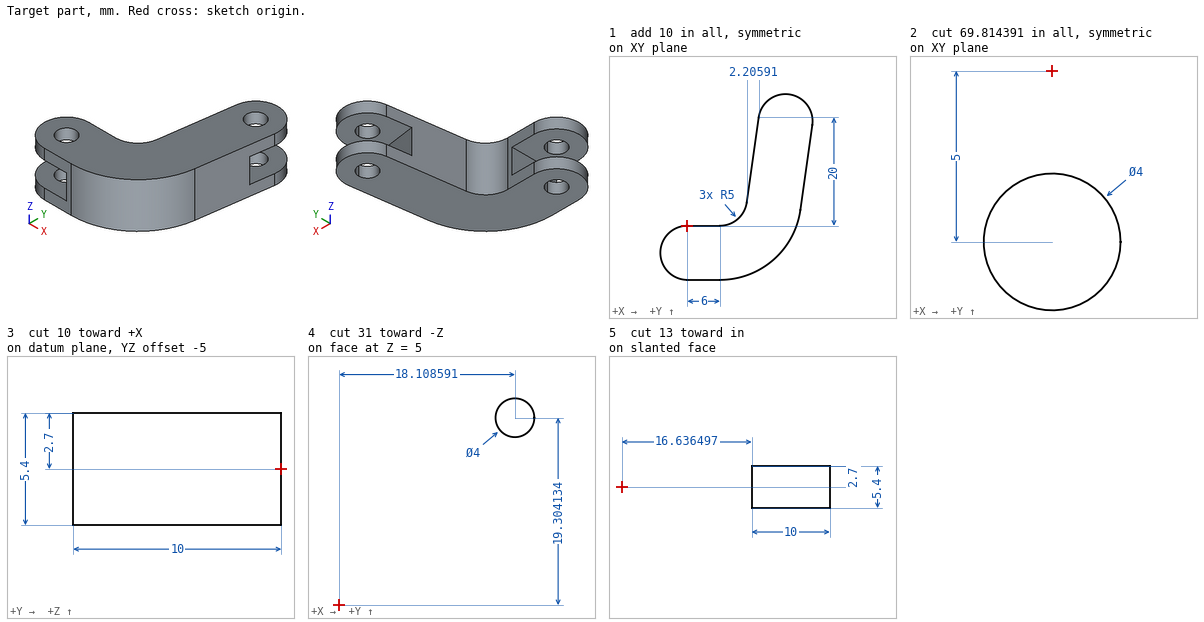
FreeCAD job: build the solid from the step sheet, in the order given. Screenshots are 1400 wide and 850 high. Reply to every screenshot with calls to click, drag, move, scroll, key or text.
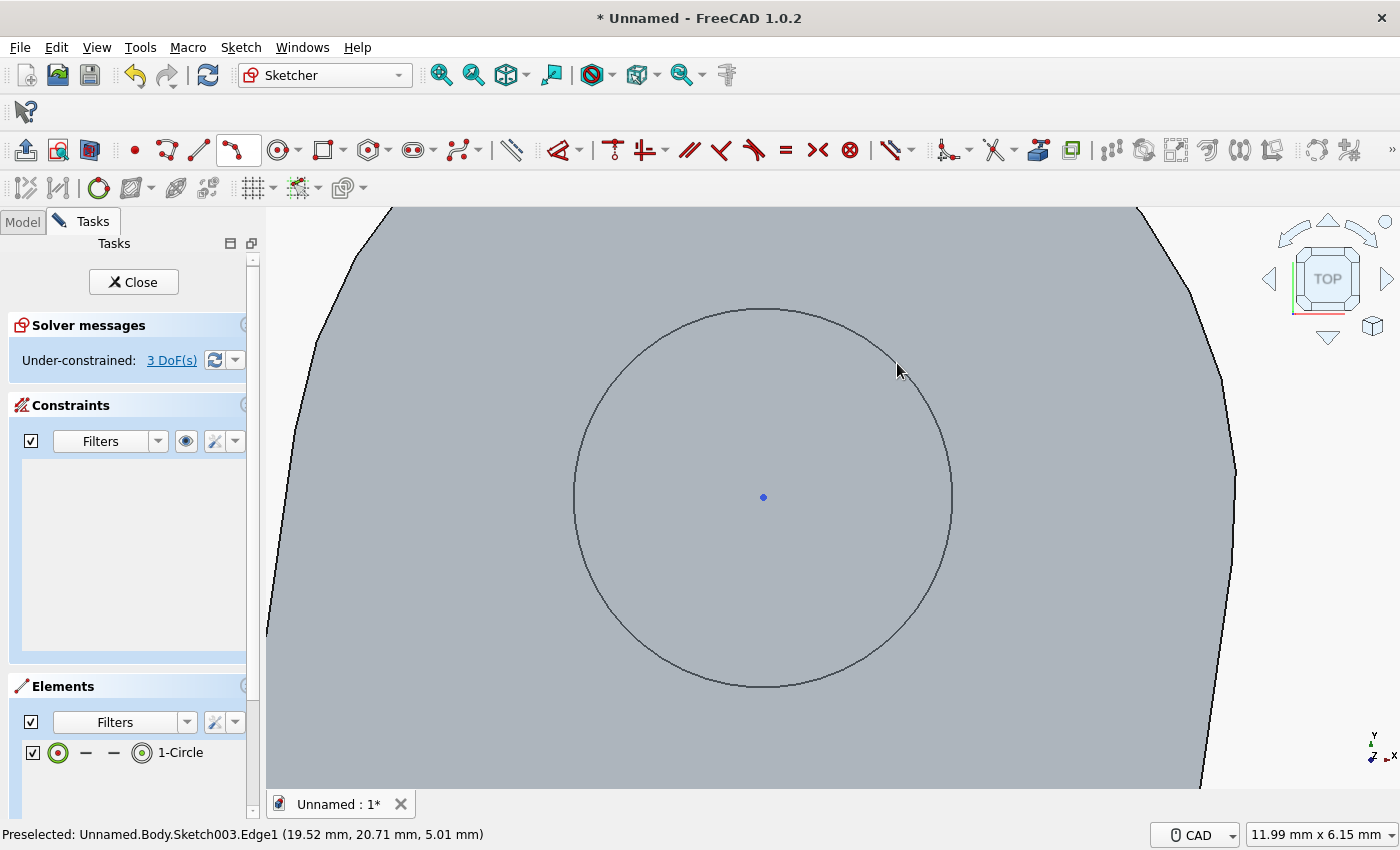
key(d)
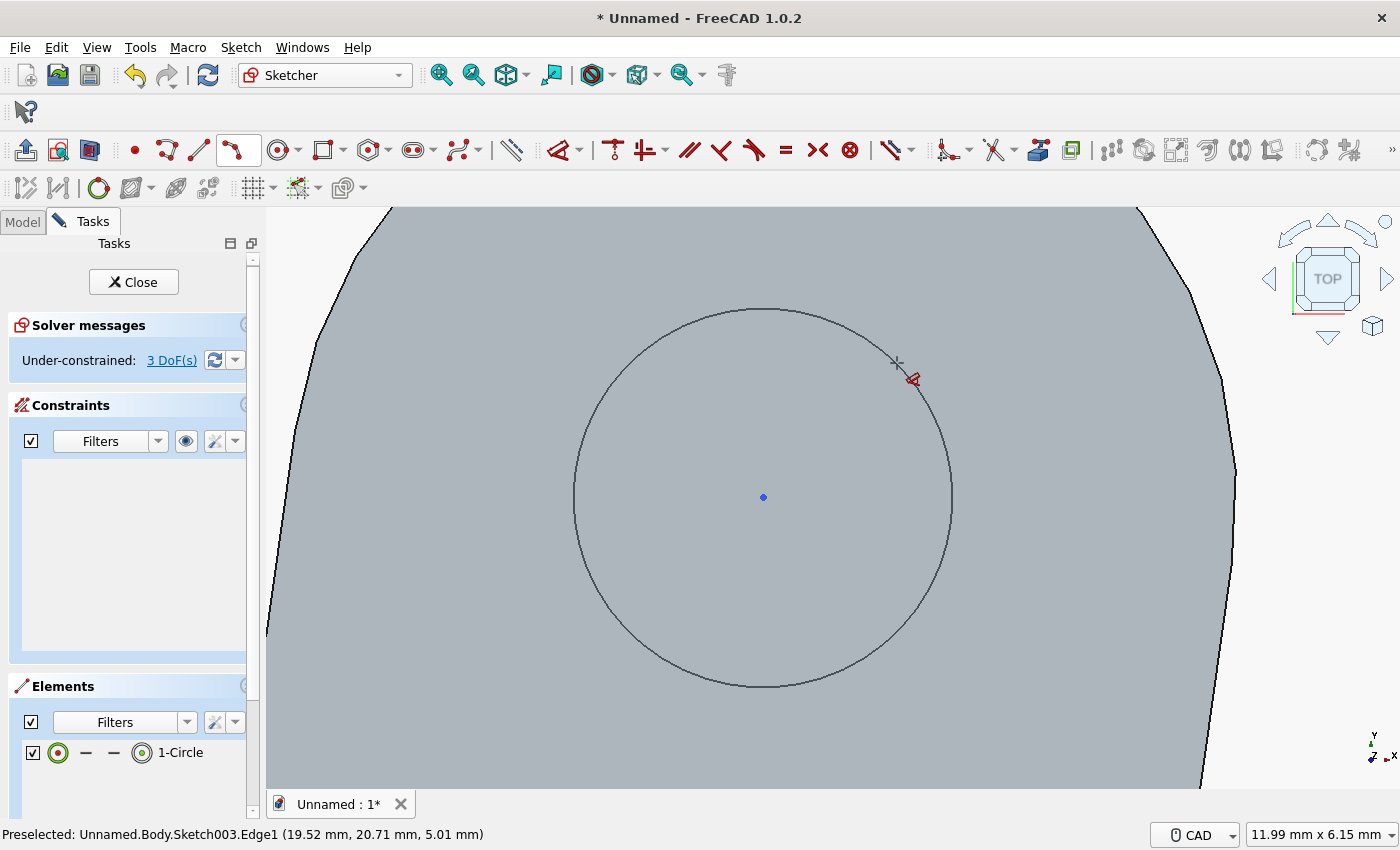
click(897, 364)
click(920, 341)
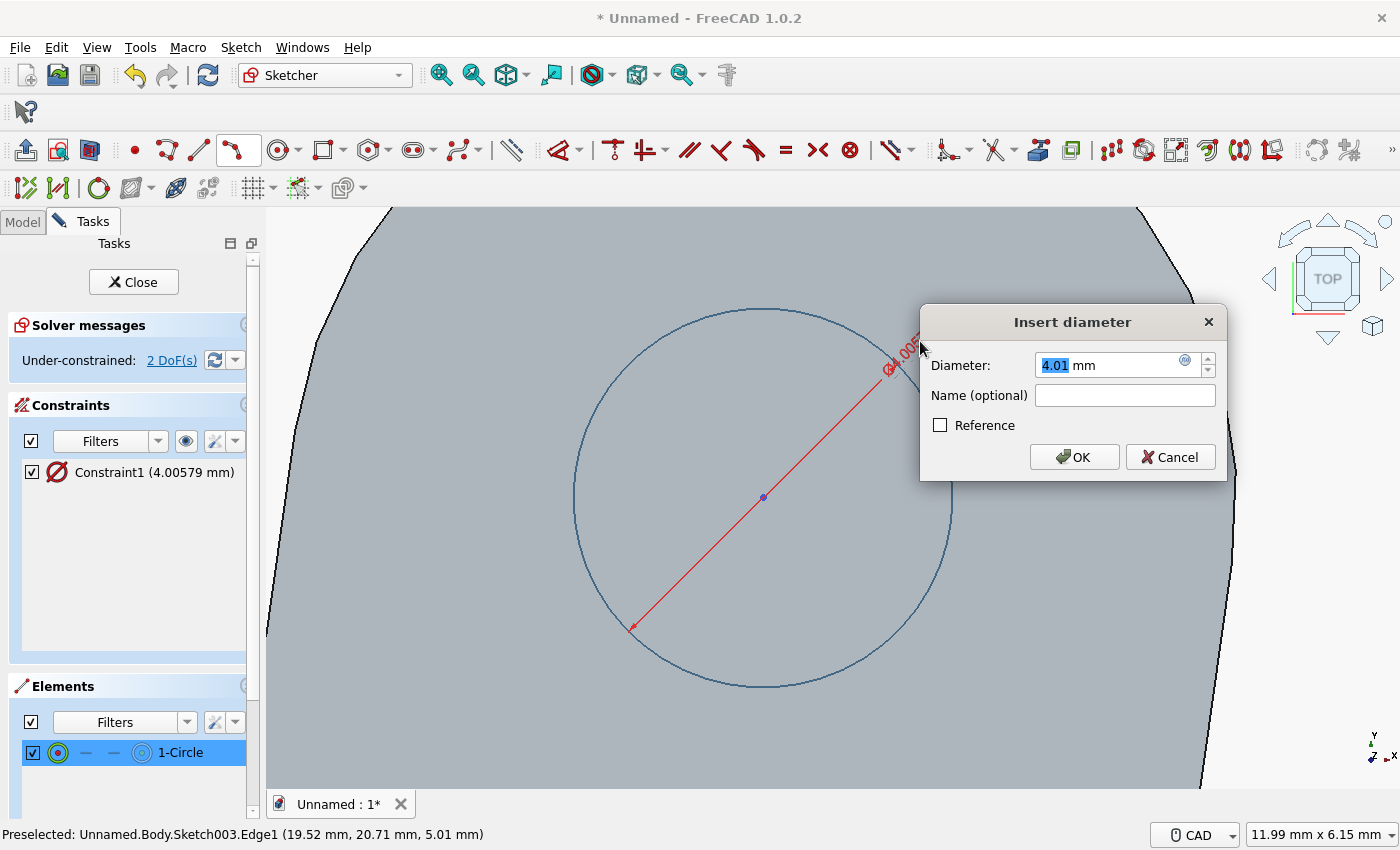
text(4)
key(Return)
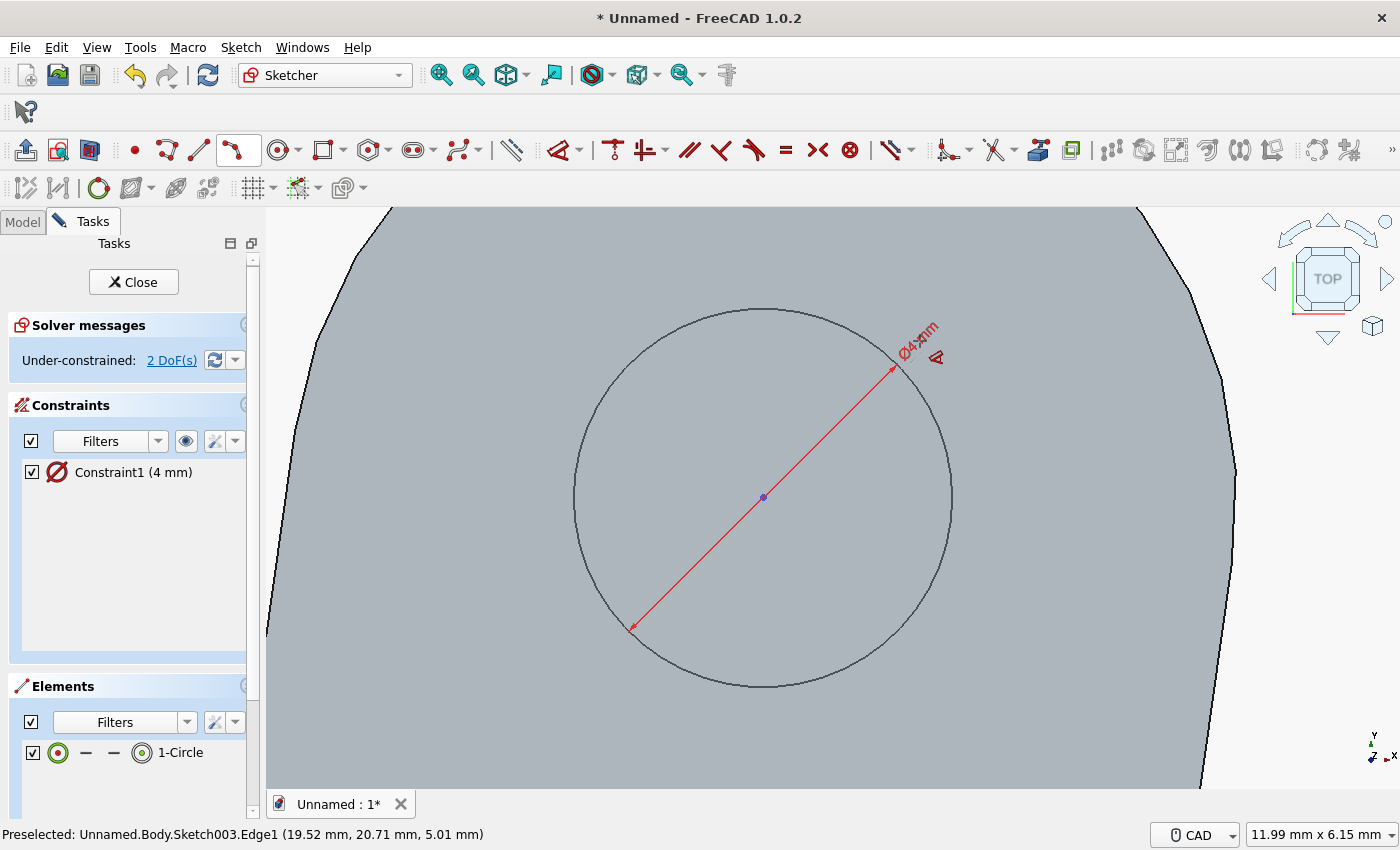
click(763, 498)
click(529, 464)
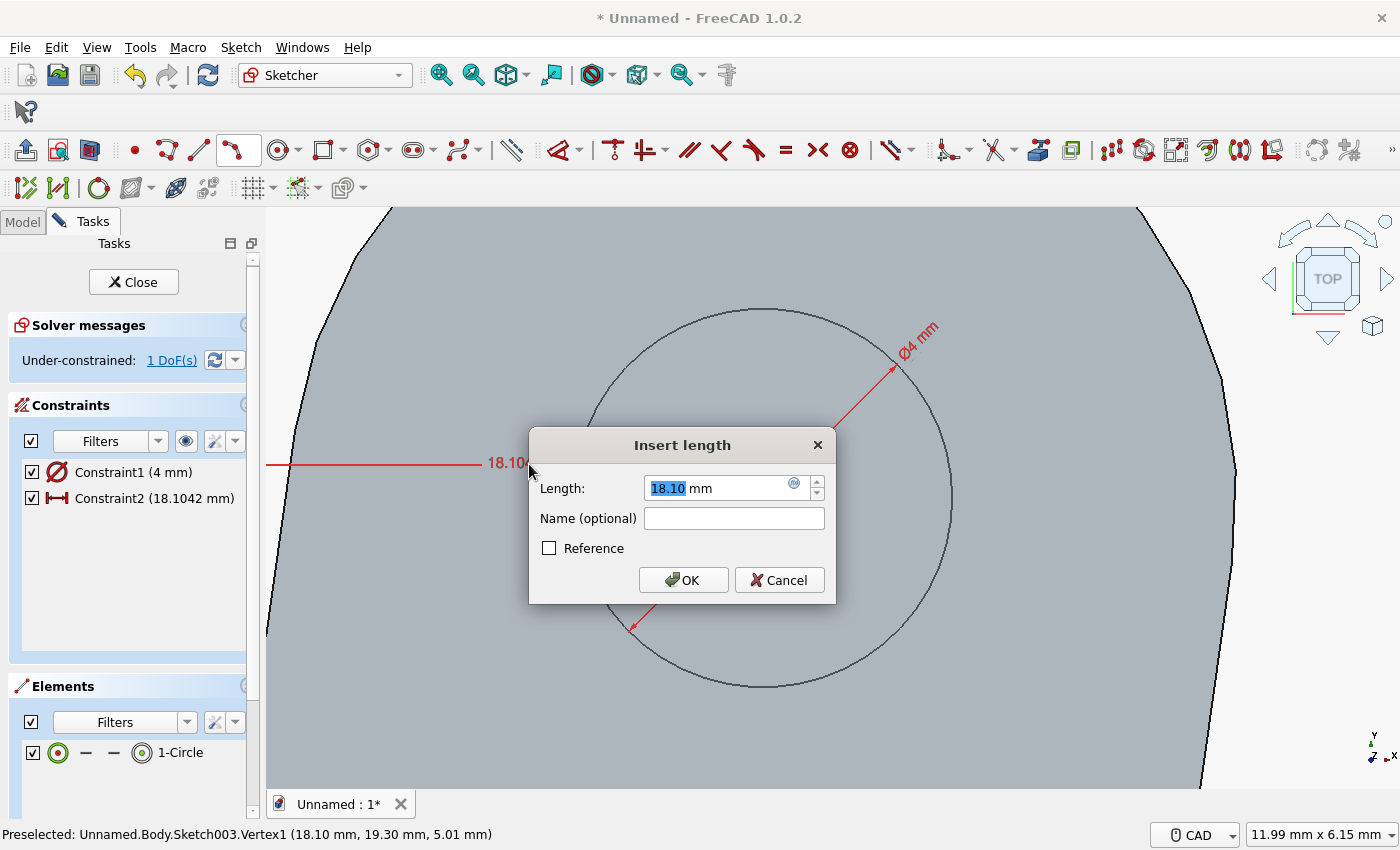
text(18.108591)
key(Return)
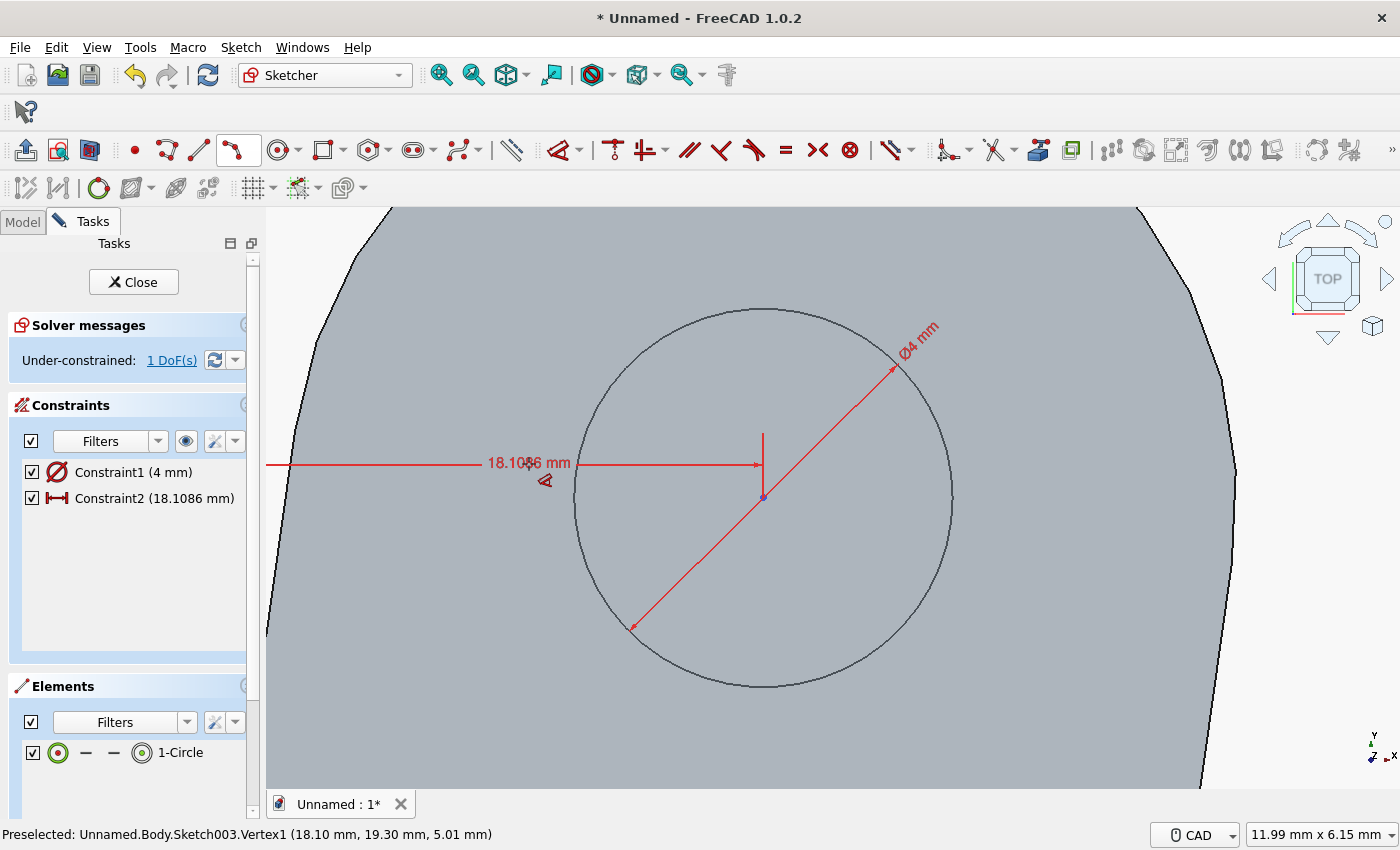
click(763, 498)
click(797, 629)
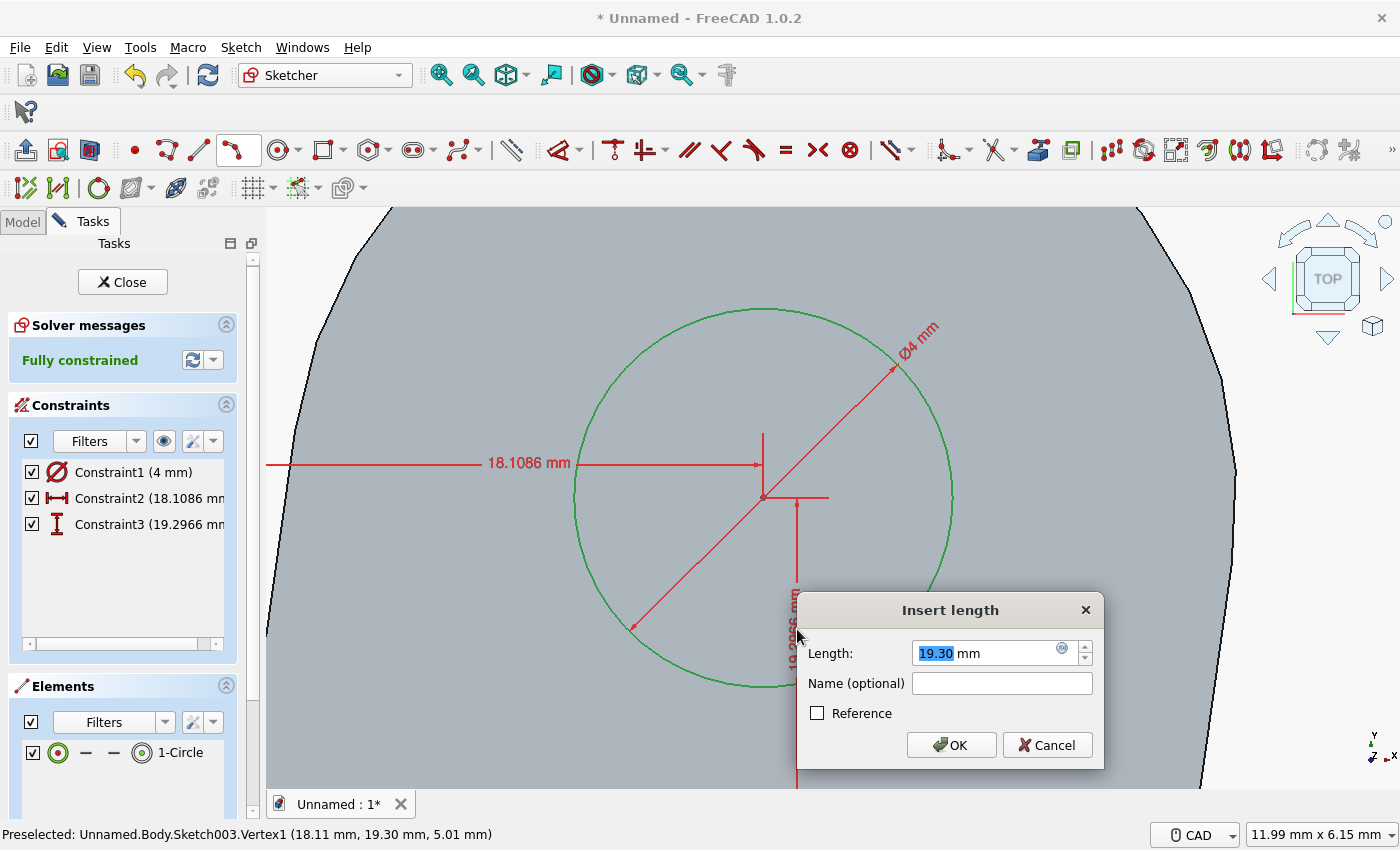
text(19.304134)
key(Return)
key(Escape)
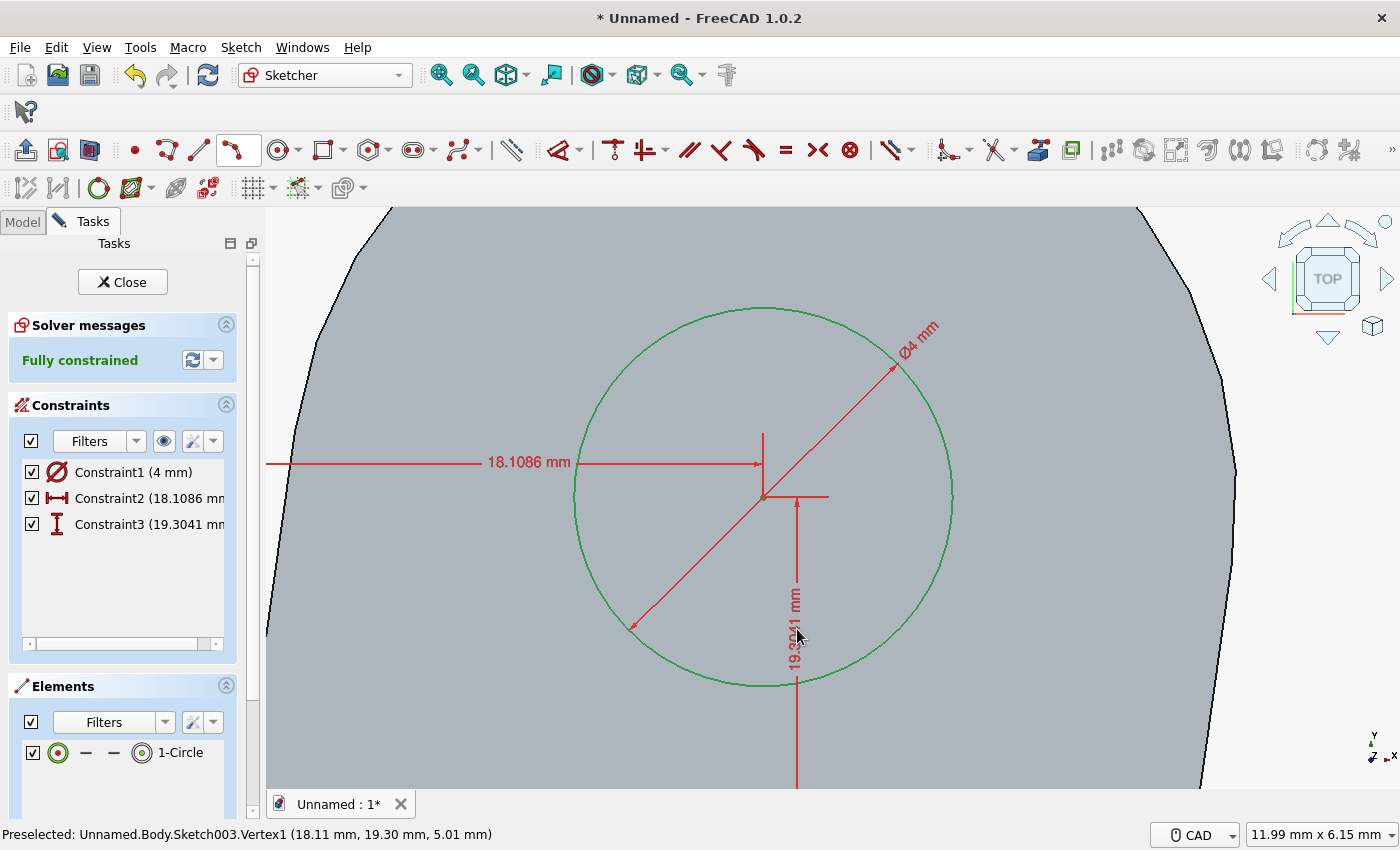
click(123, 282)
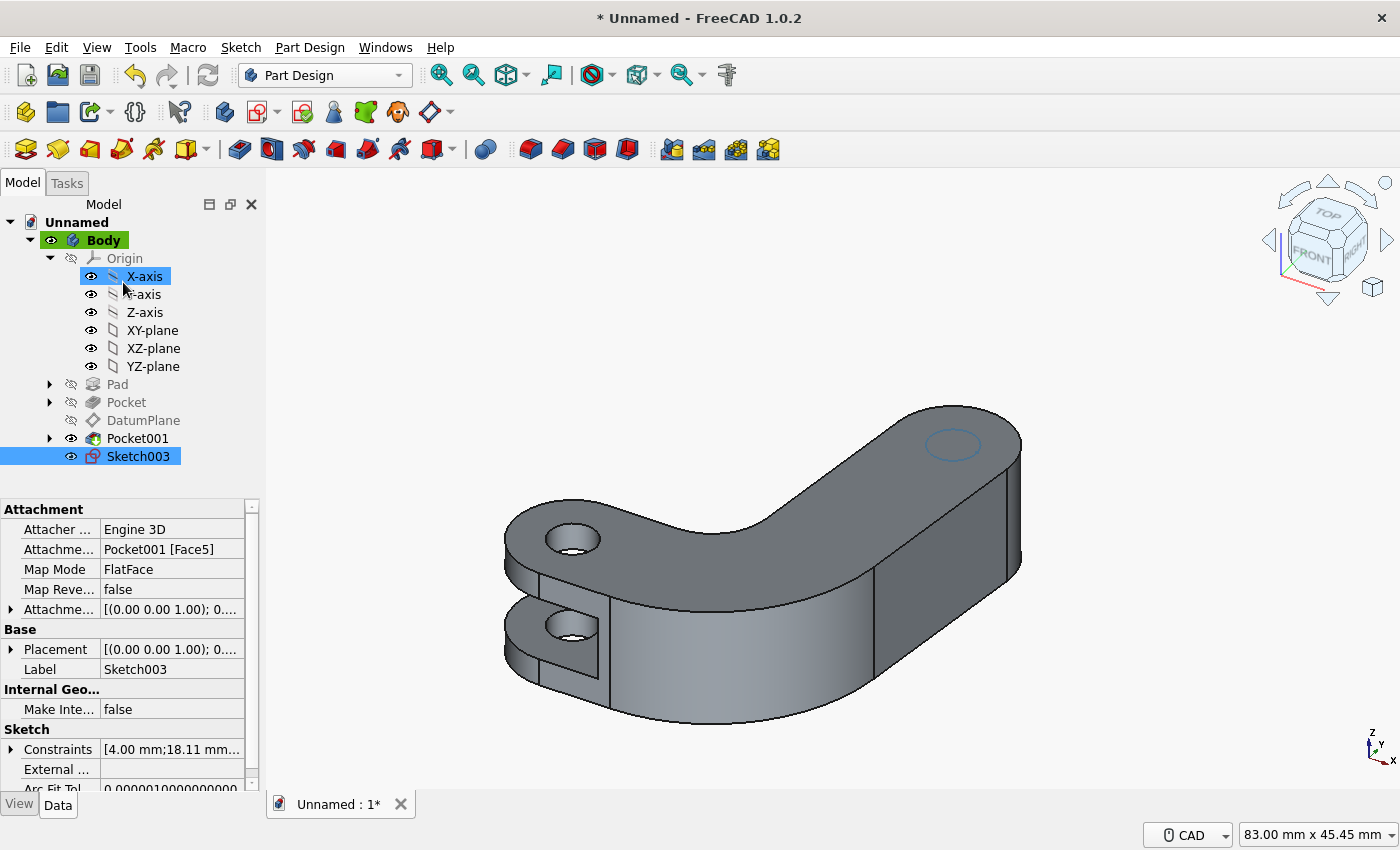
click(240, 150)